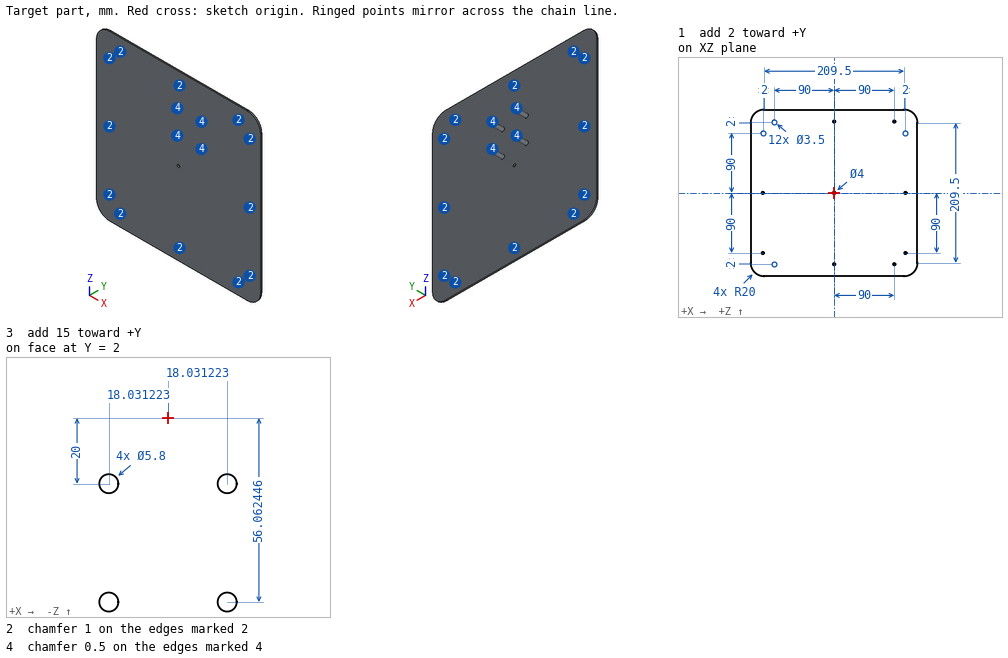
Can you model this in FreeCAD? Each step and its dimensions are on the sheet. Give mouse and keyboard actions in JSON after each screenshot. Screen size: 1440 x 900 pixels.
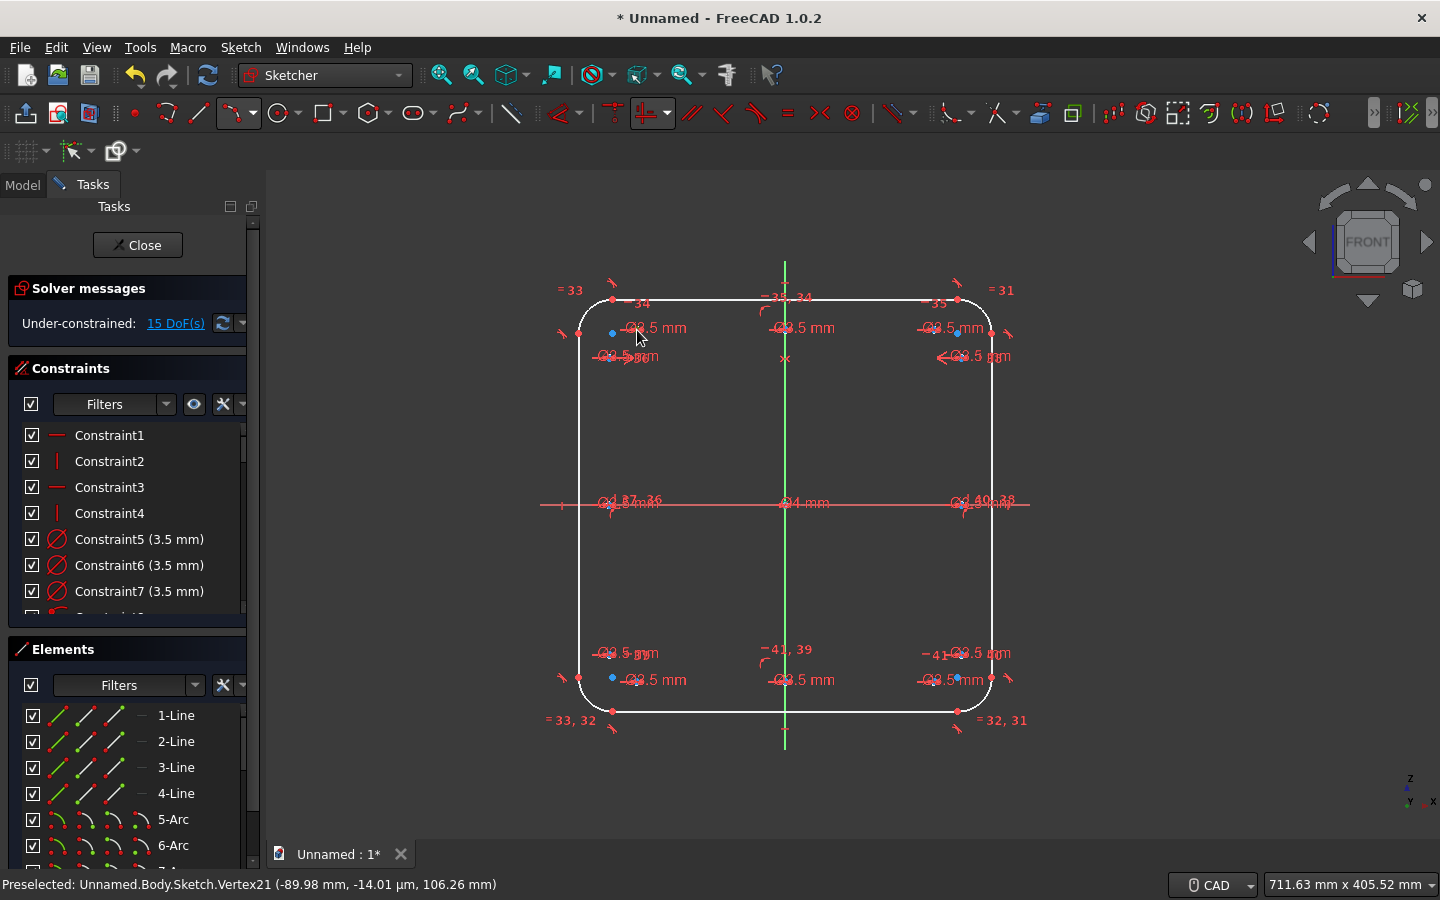
{"action": "left_click", "coordinate": [637, 682]}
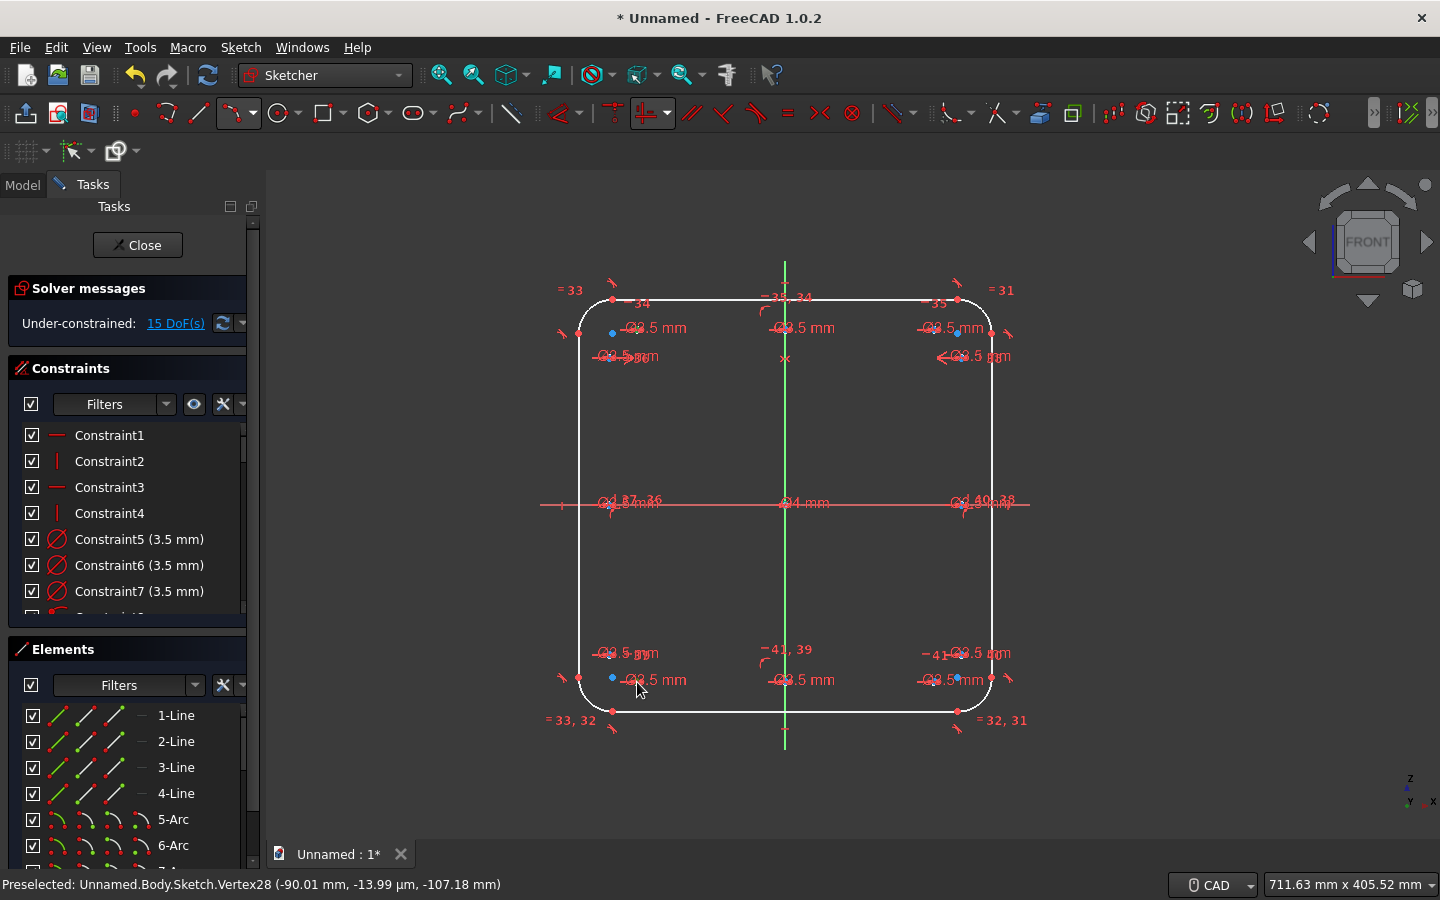
{"action": "left_click", "coordinate": [714, 505]}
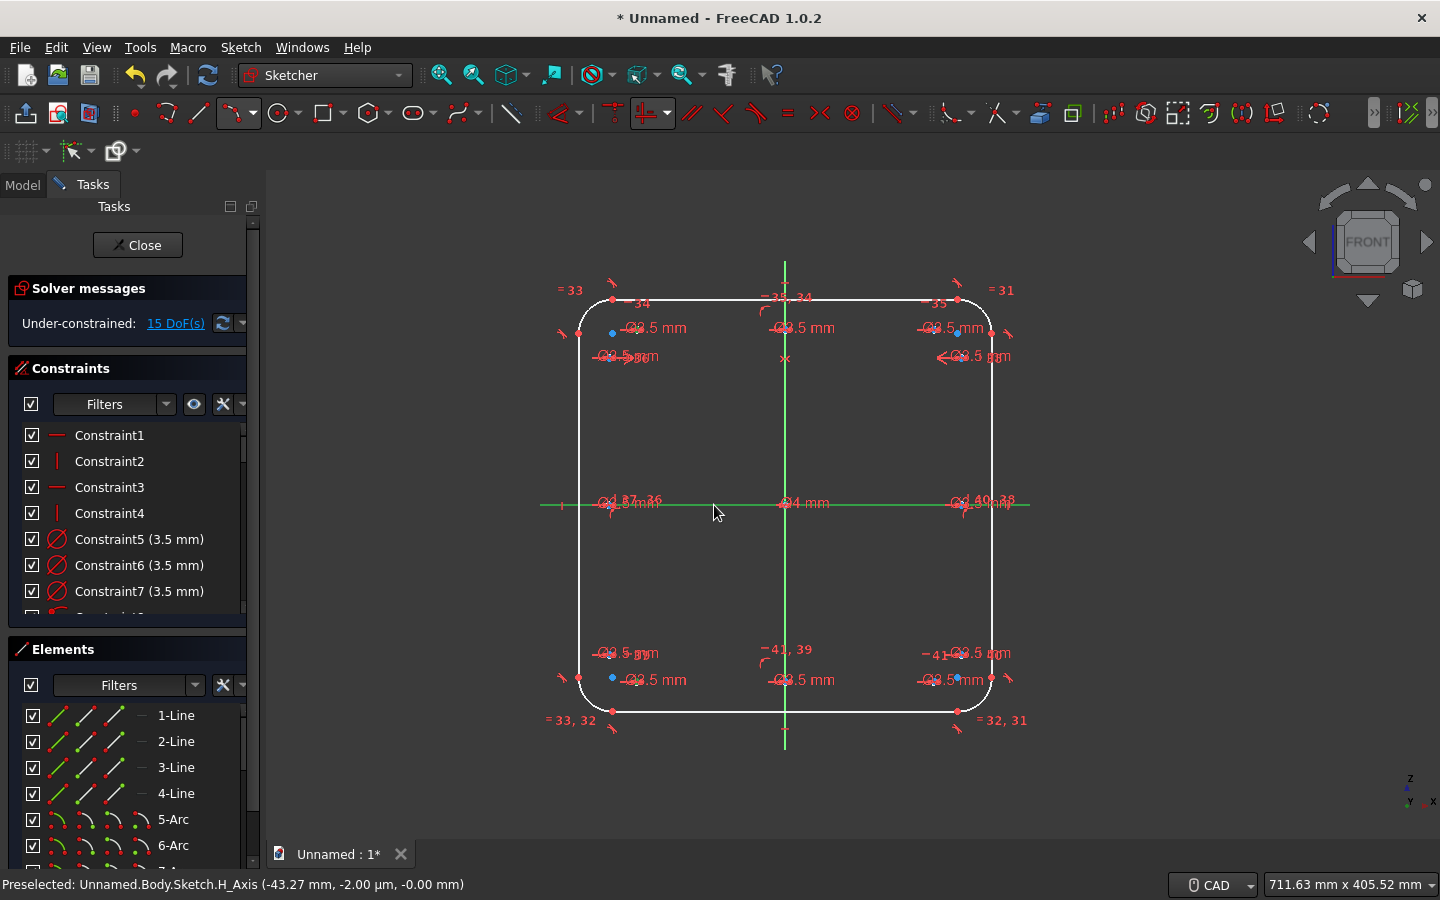
{"action": "left_click", "coordinate": [820, 114]}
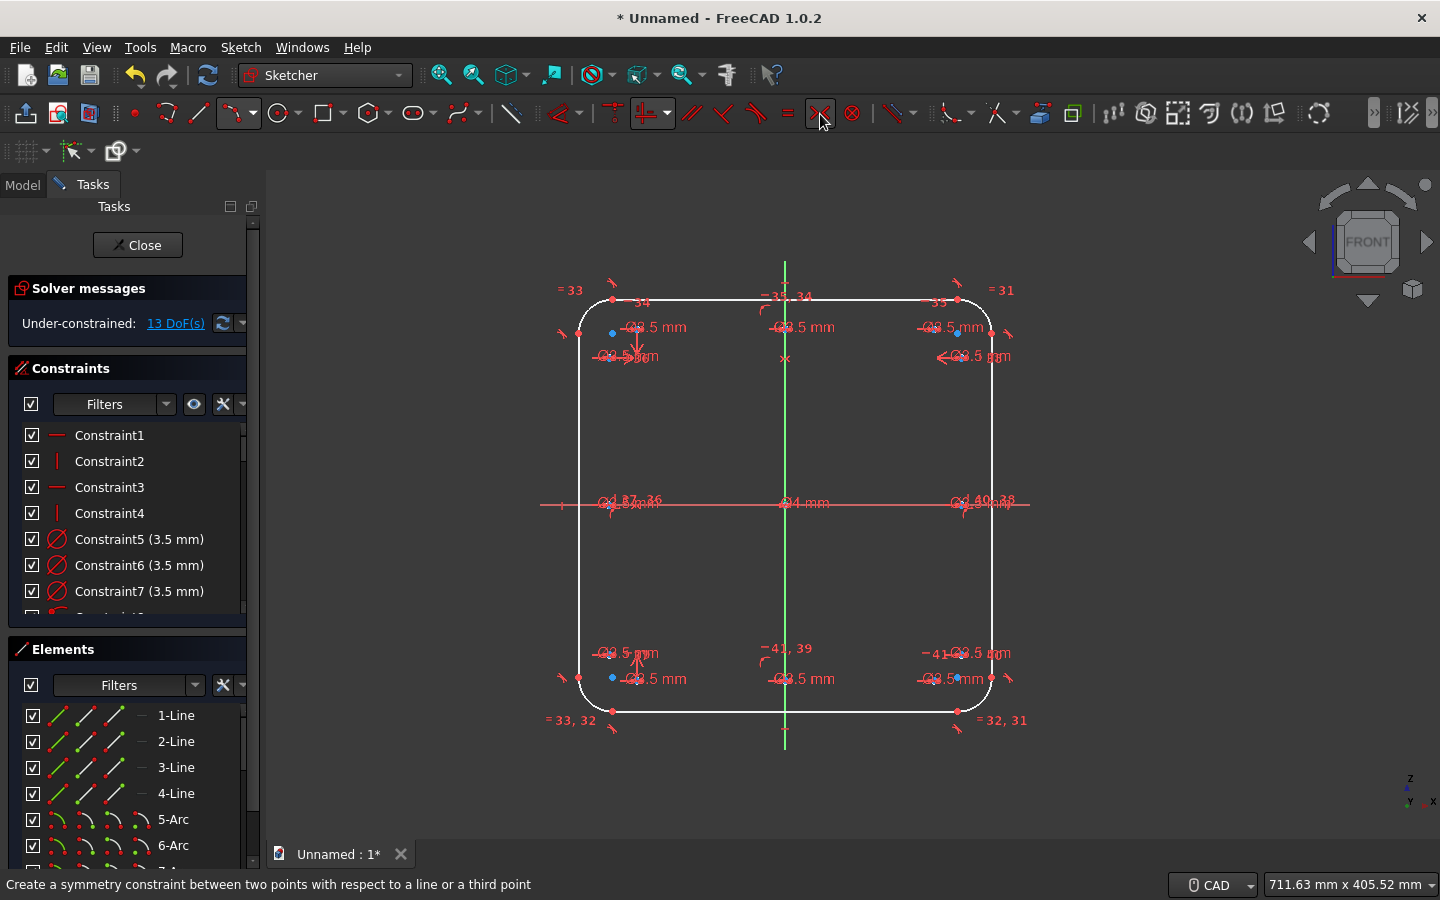
{"action": "key", "text": "d"}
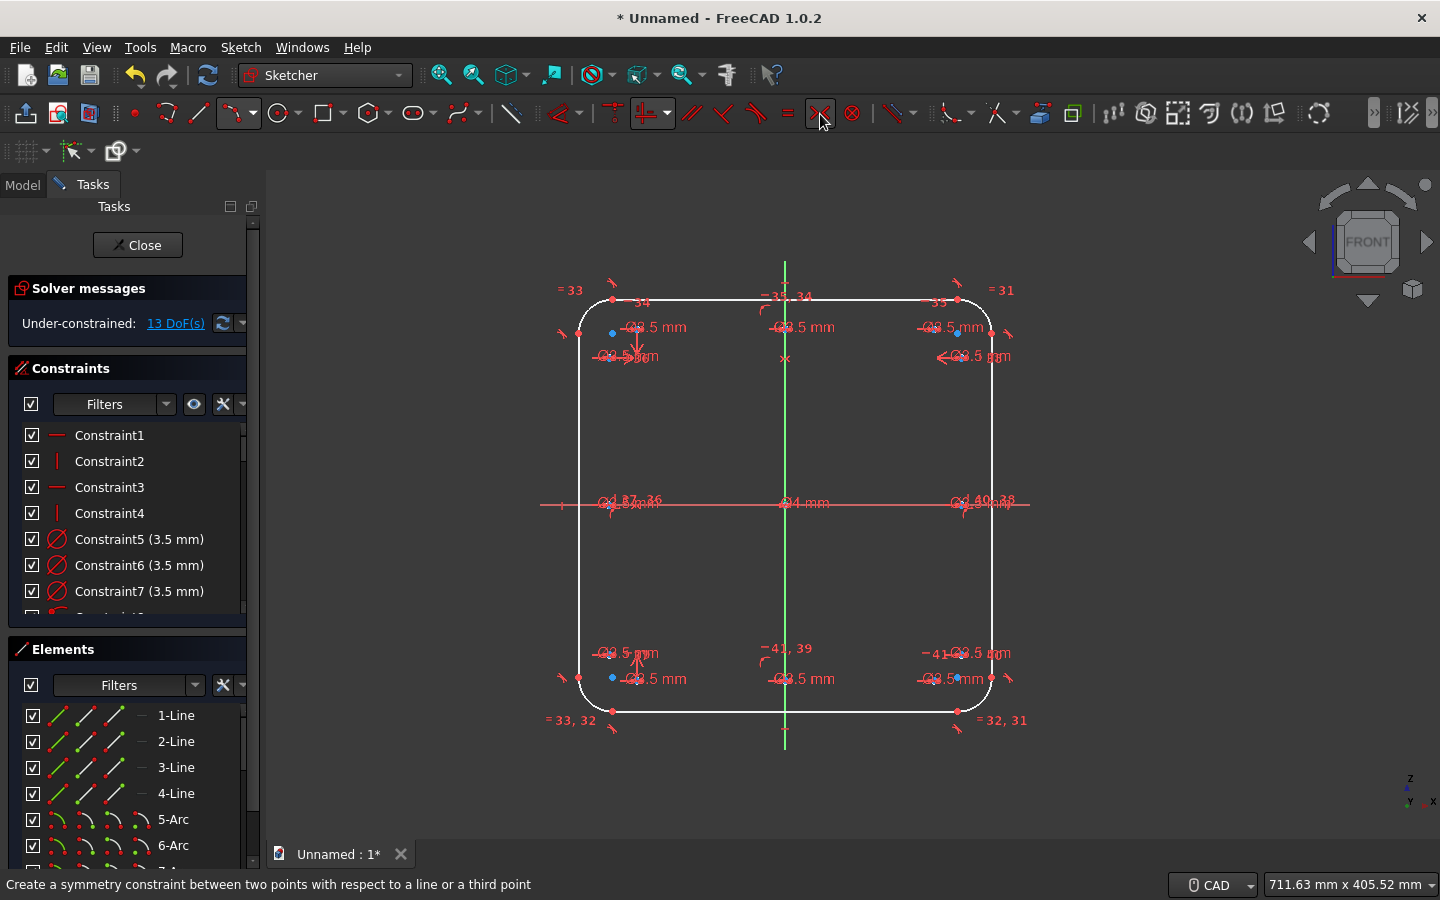
{"action": "left_click", "coordinate": [988, 318]}
{"action": "left_click", "coordinate": [1016, 303]}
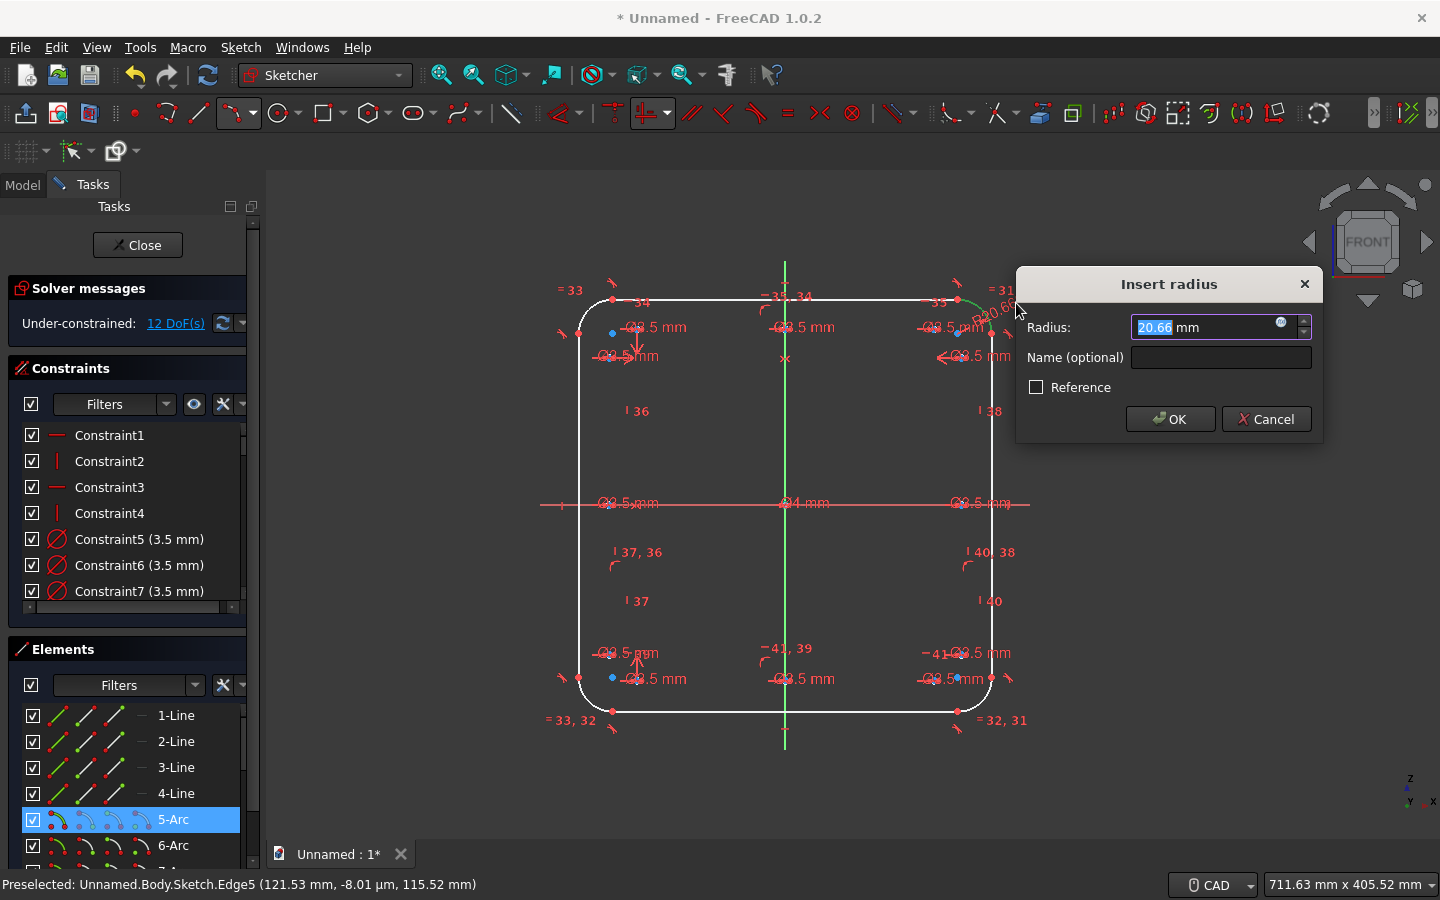
{"action": "type", "text": "20"}
{"action": "key", "text": "Return"}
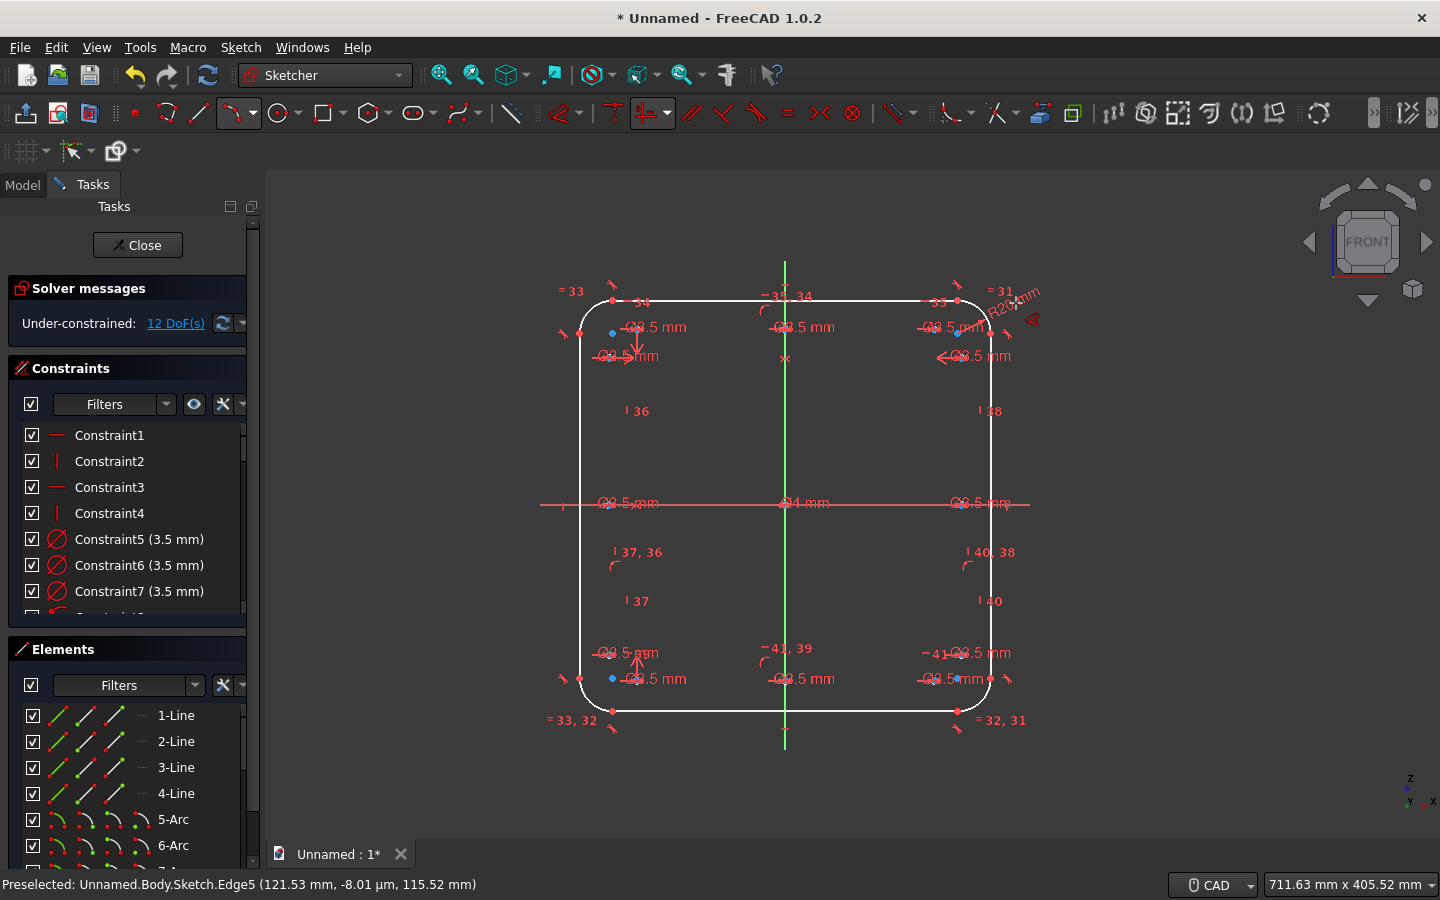
{"action": "left_click", "coordinate": [637, 329]}
{"action": "left_click", "coordinate": [711, 539]}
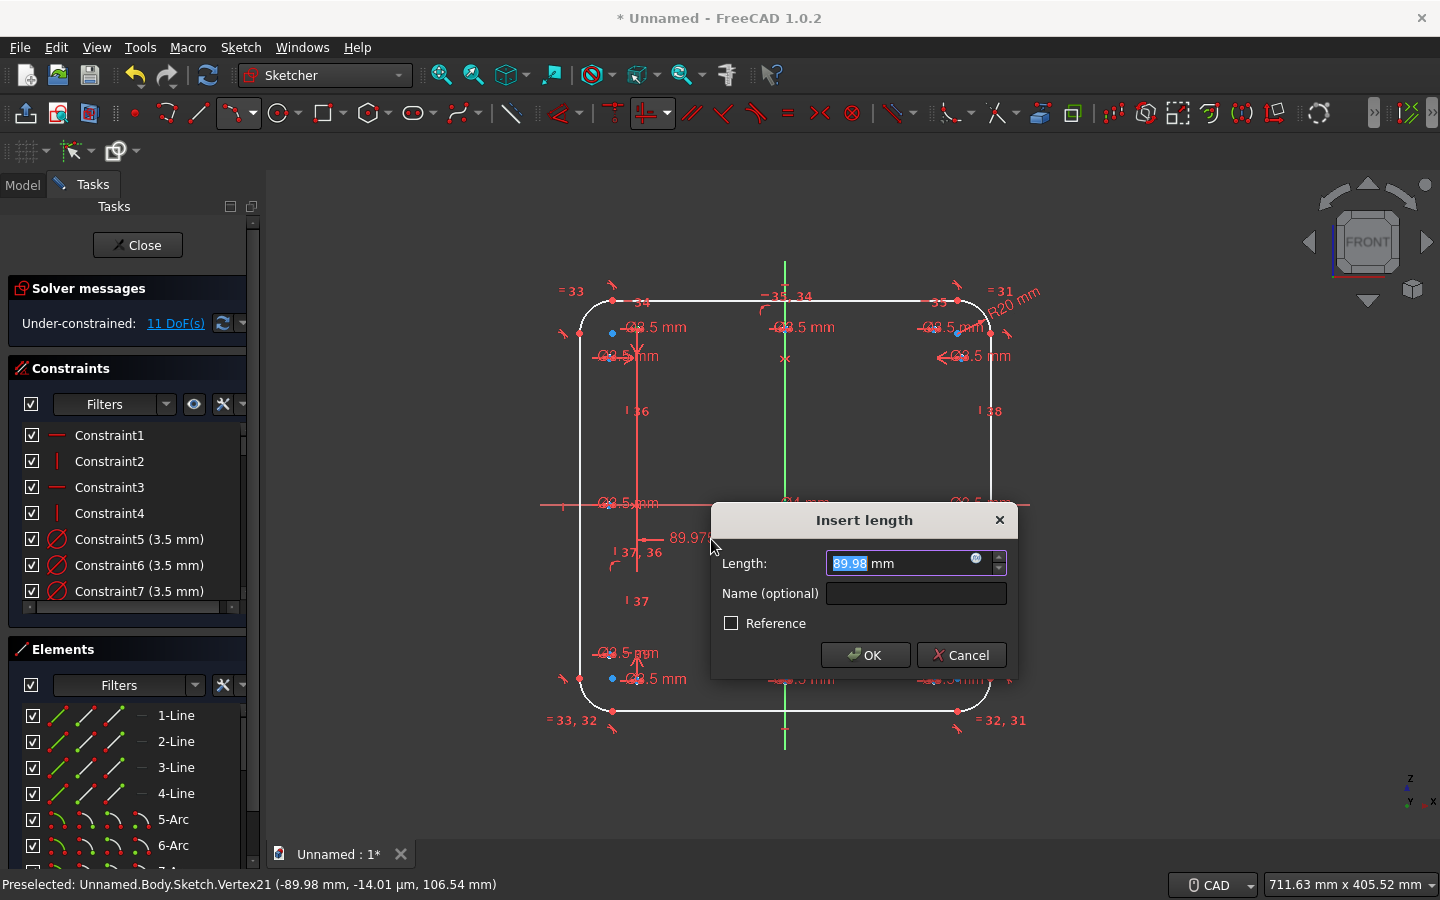
{"action": "type", "text": "90"}
{"action": "key", "text": "Return"}